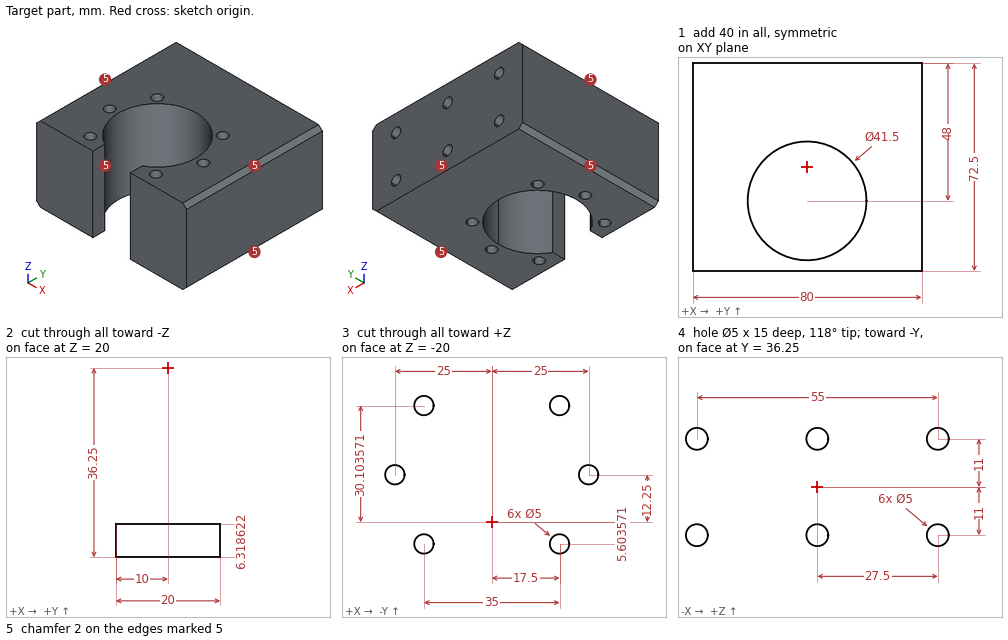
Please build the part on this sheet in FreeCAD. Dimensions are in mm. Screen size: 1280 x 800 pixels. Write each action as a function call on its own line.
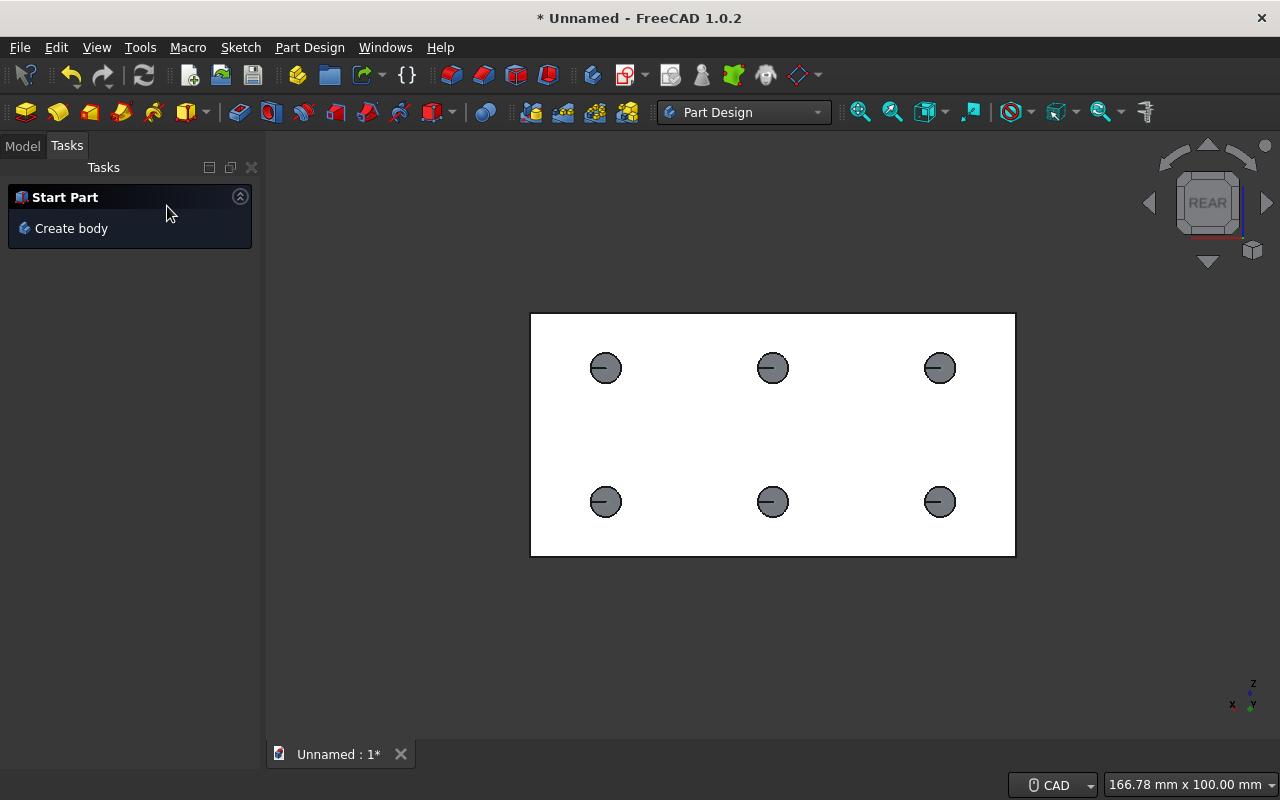
key(0)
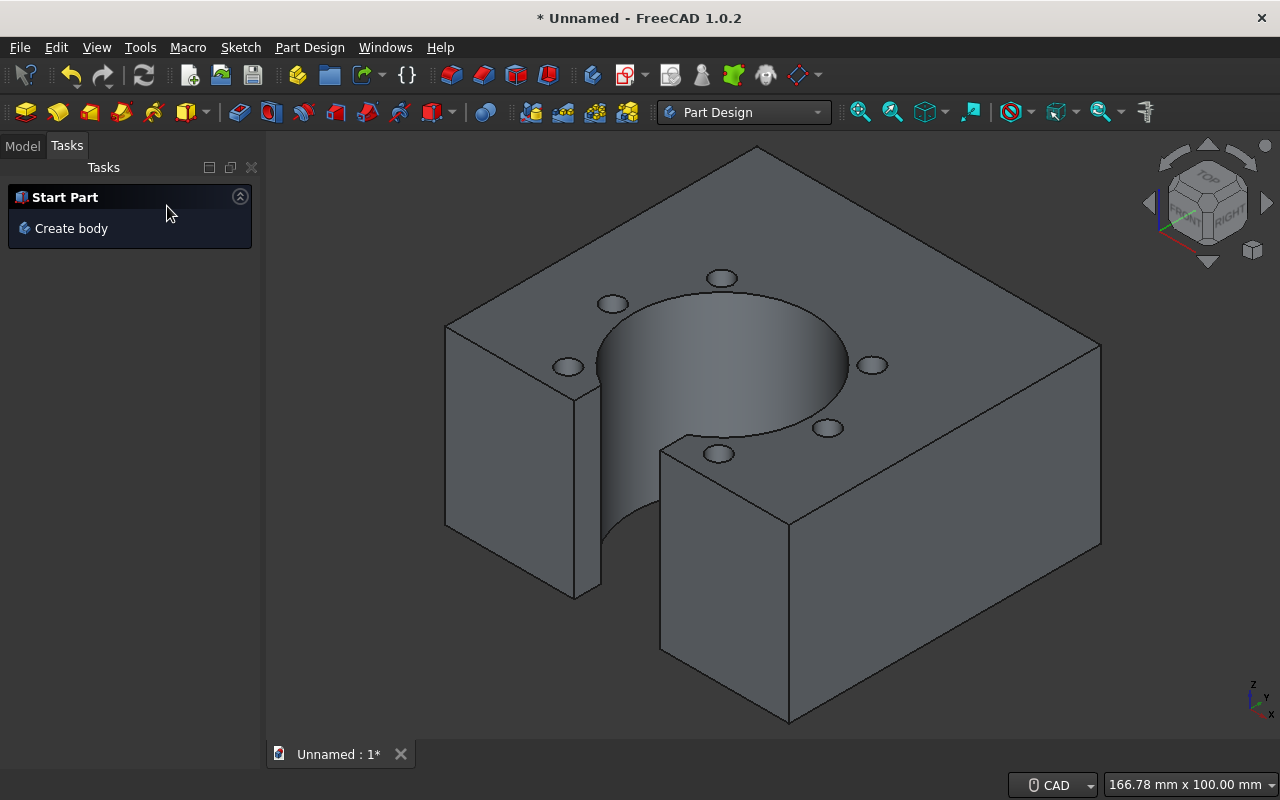
click(945, 434)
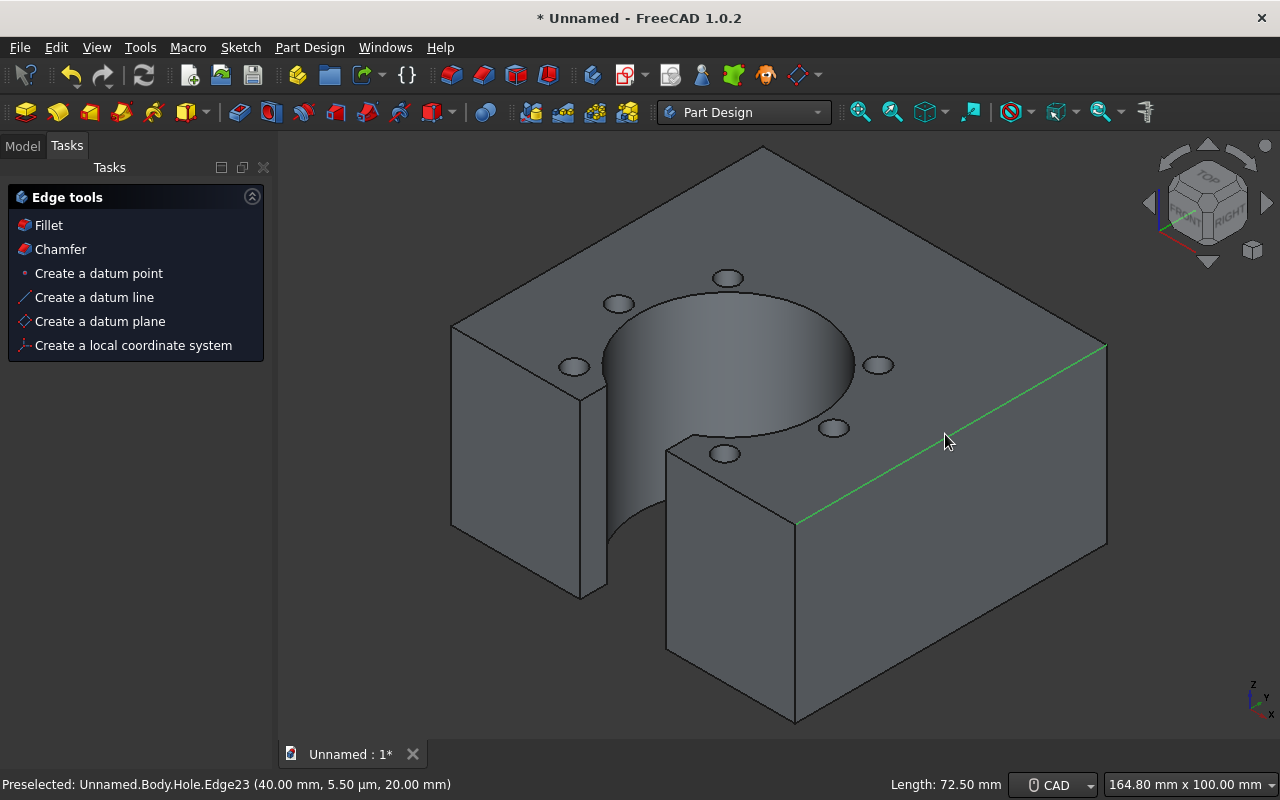
key(2)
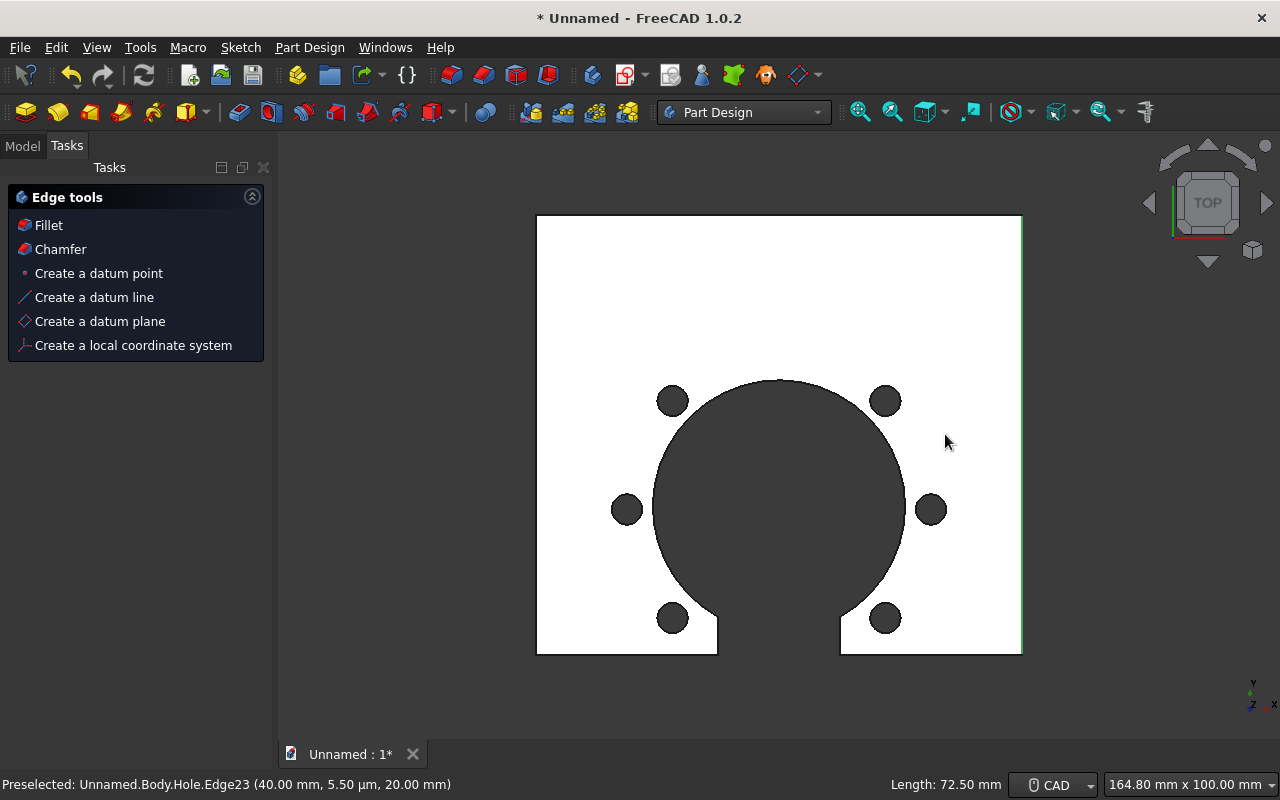
click(536, 434, ctrl)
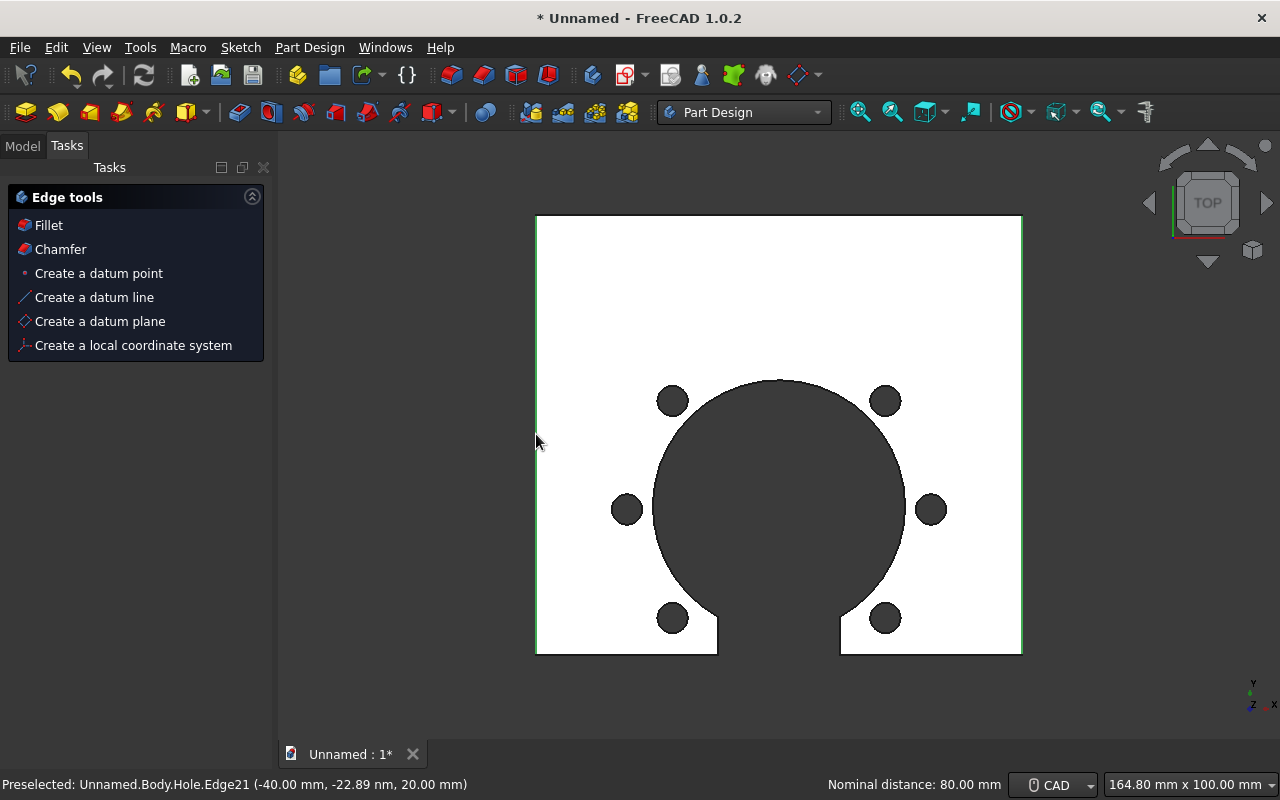
key(1)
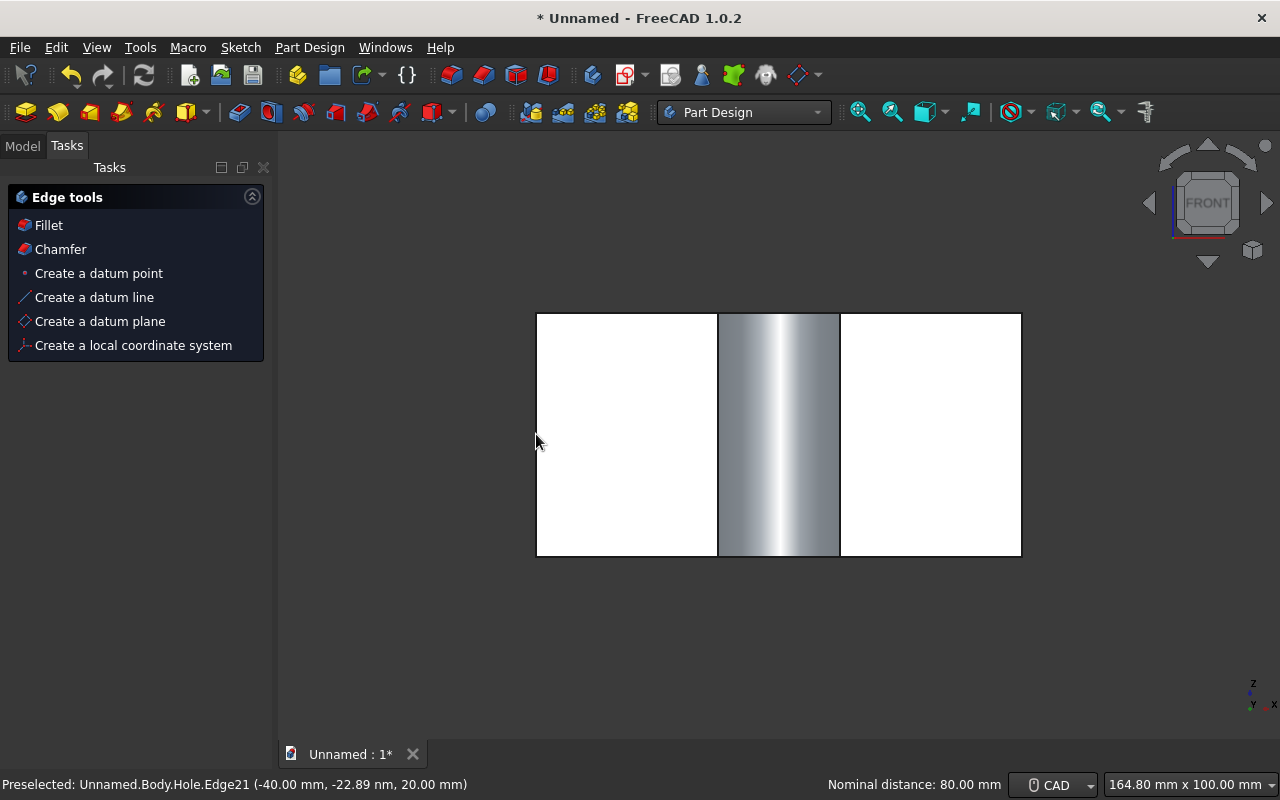
key(3)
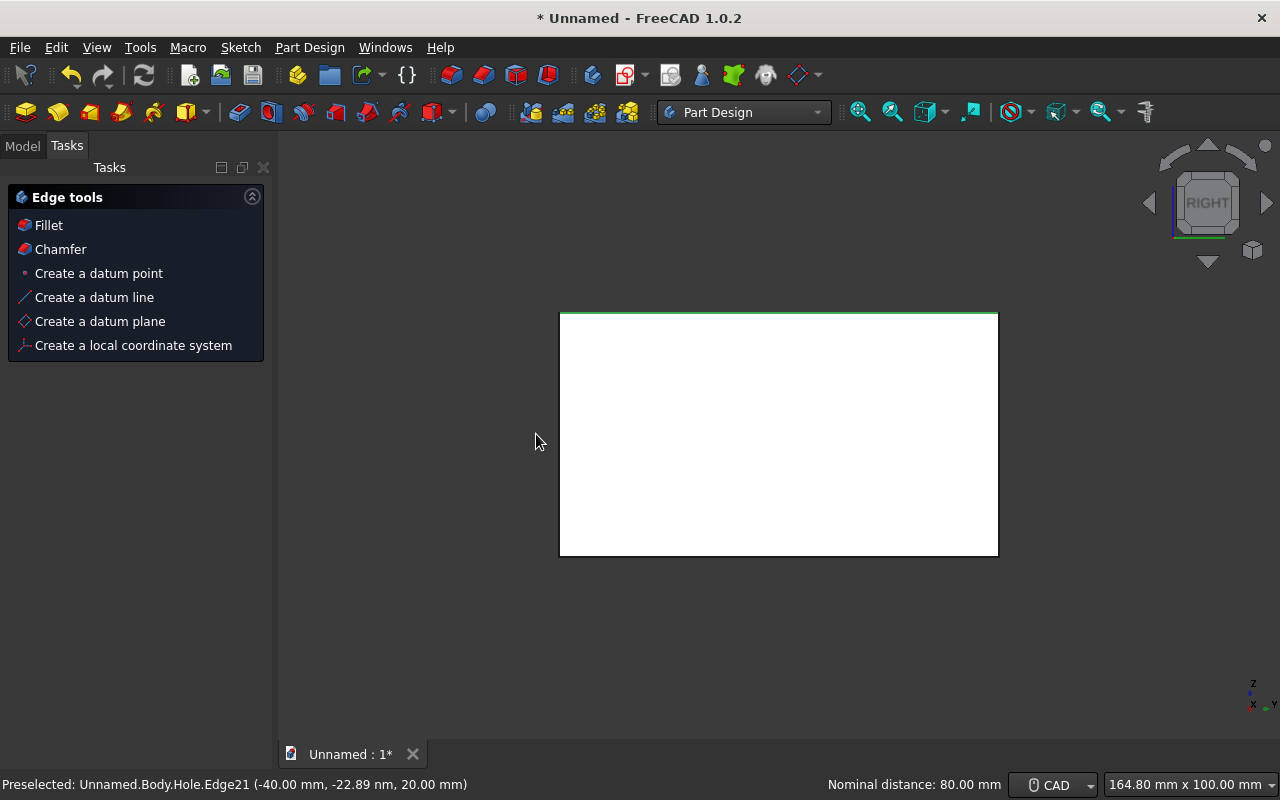
key(v)
key(f)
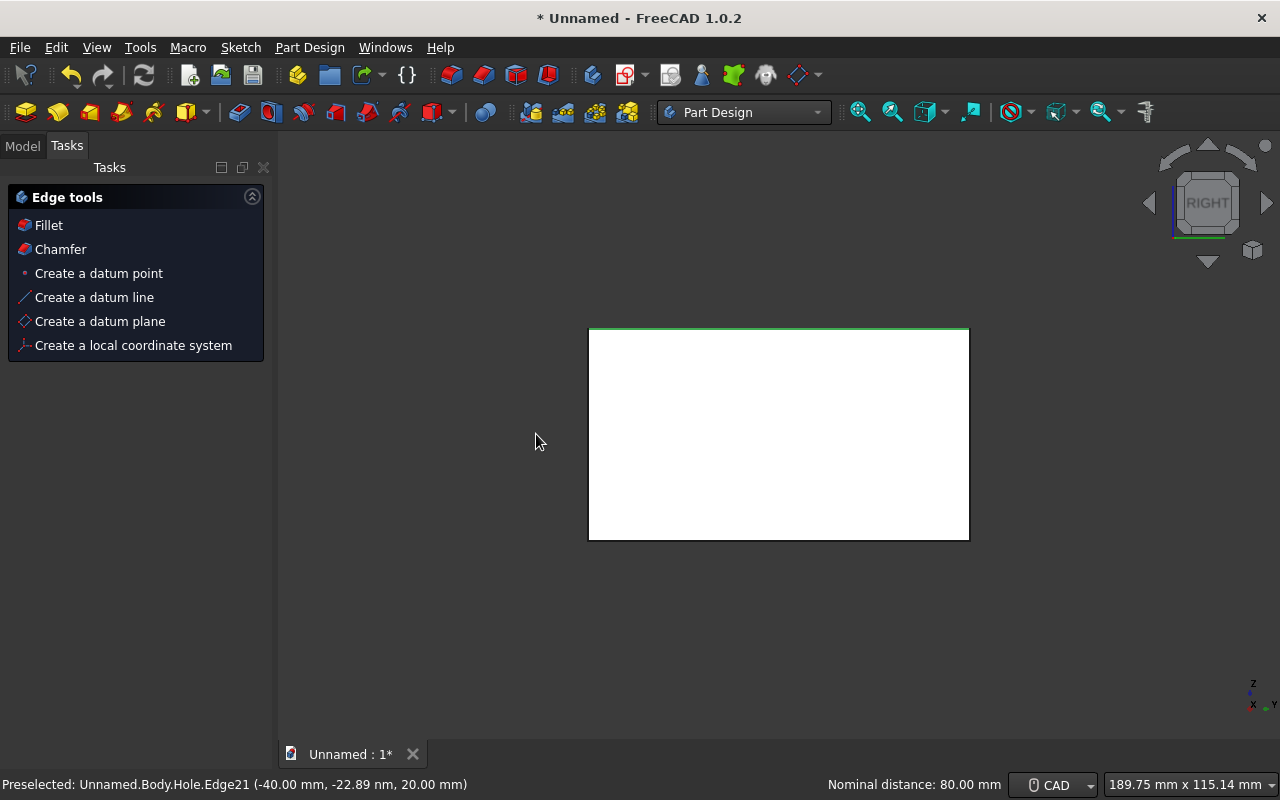
click(779, 540, ctrl)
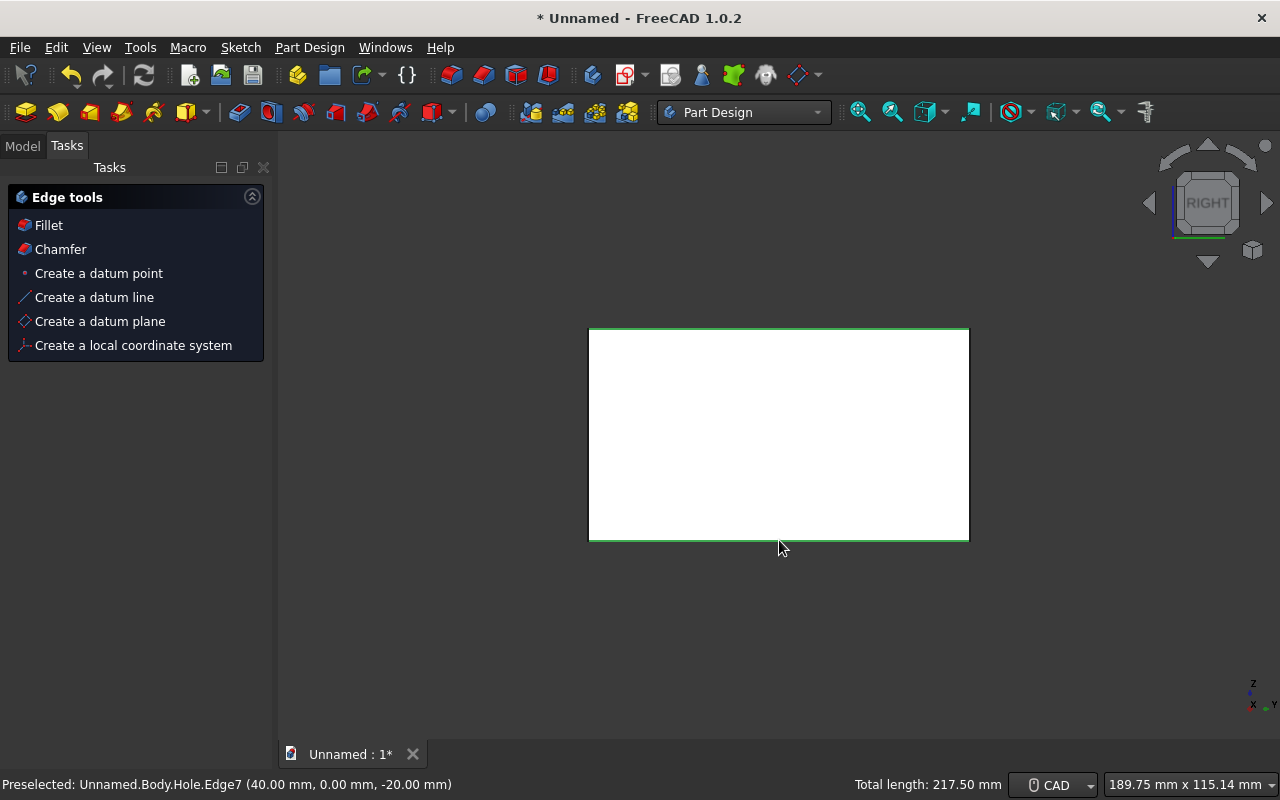
key(5)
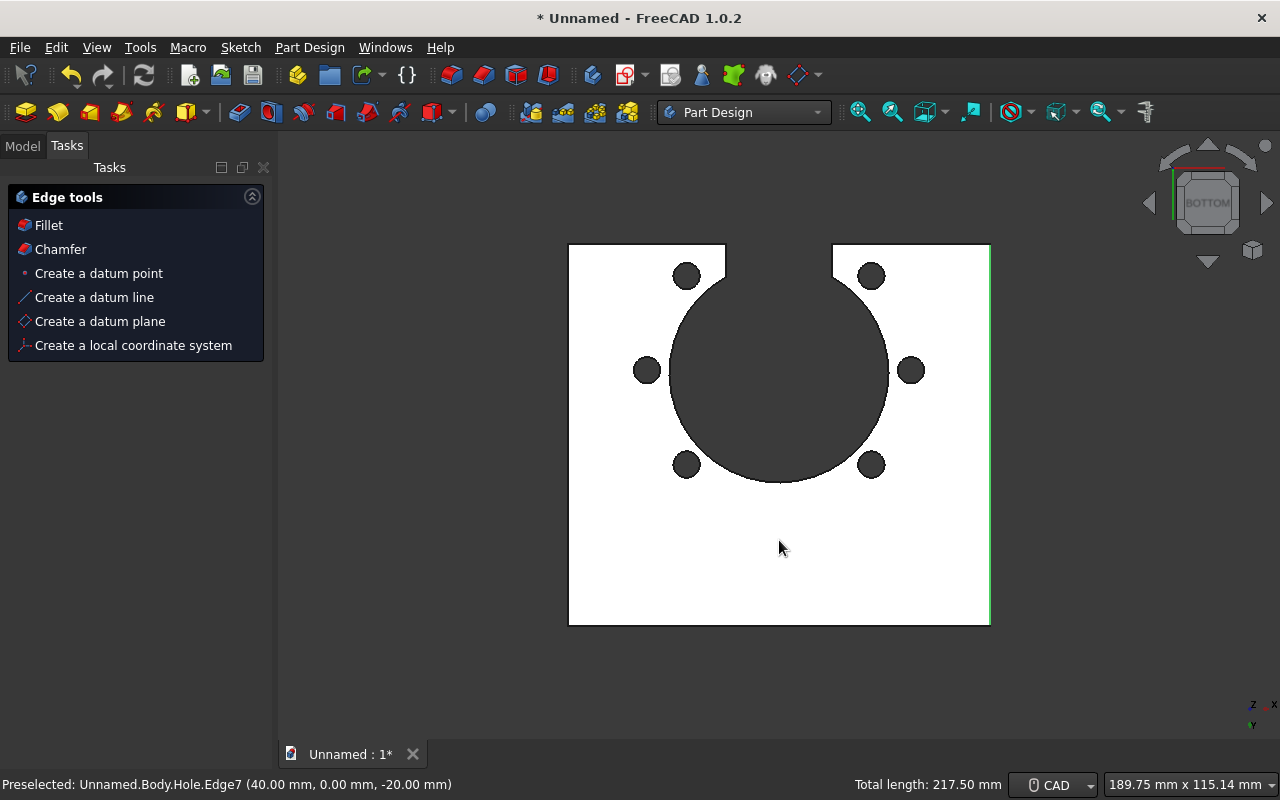
click(568, 434, ctrl)